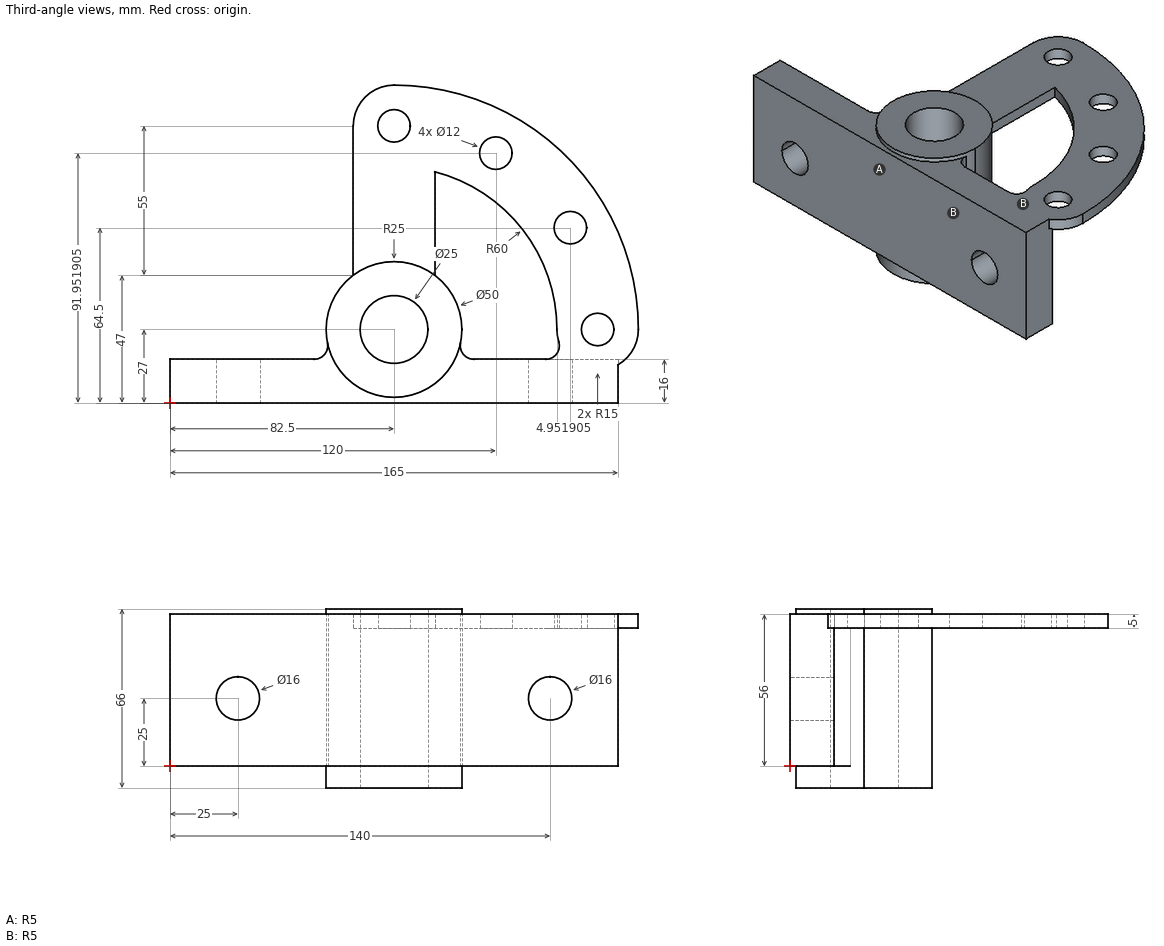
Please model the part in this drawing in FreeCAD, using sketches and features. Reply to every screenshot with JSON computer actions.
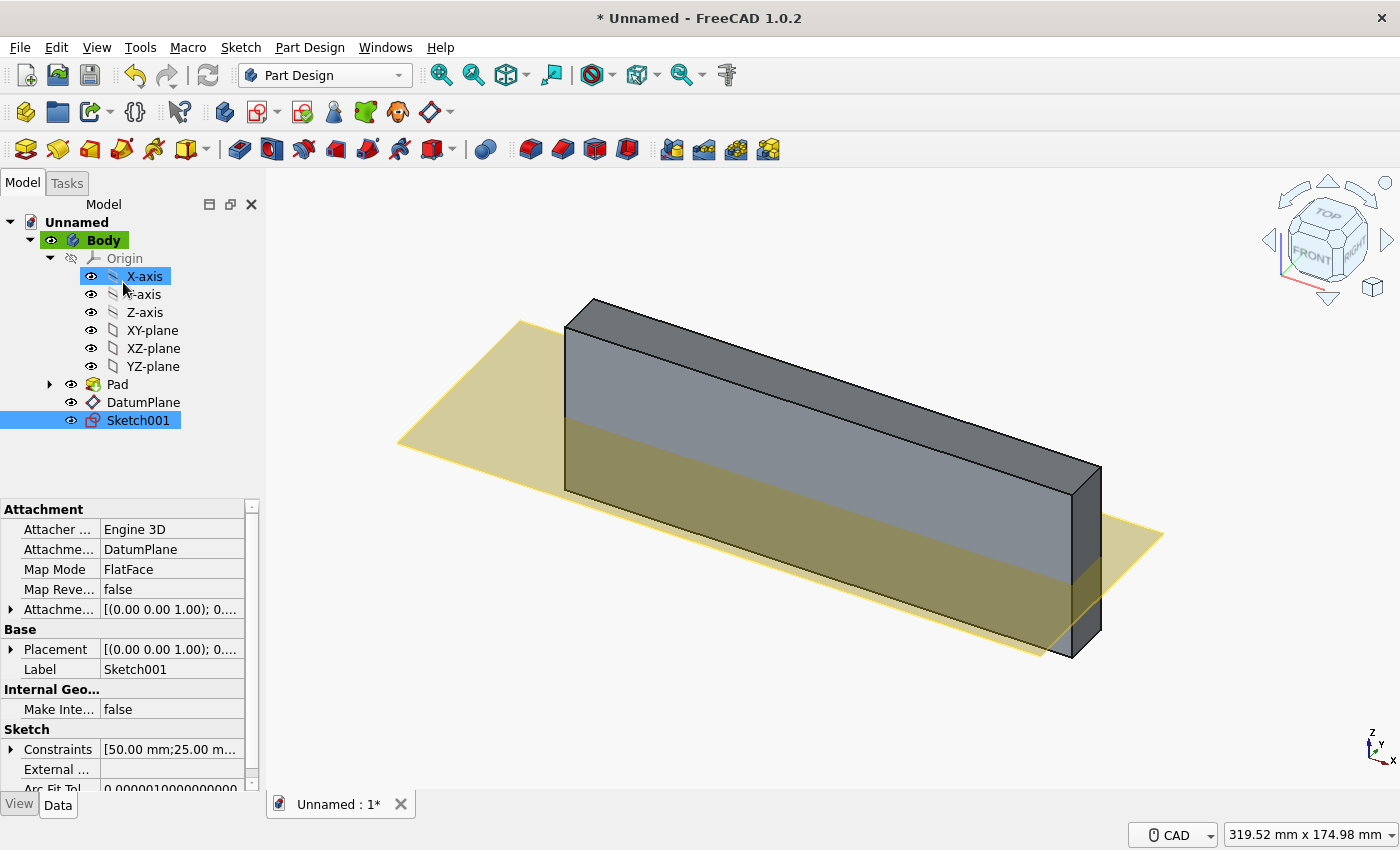
{"action": "left_click", "coordinate": [26, 150]}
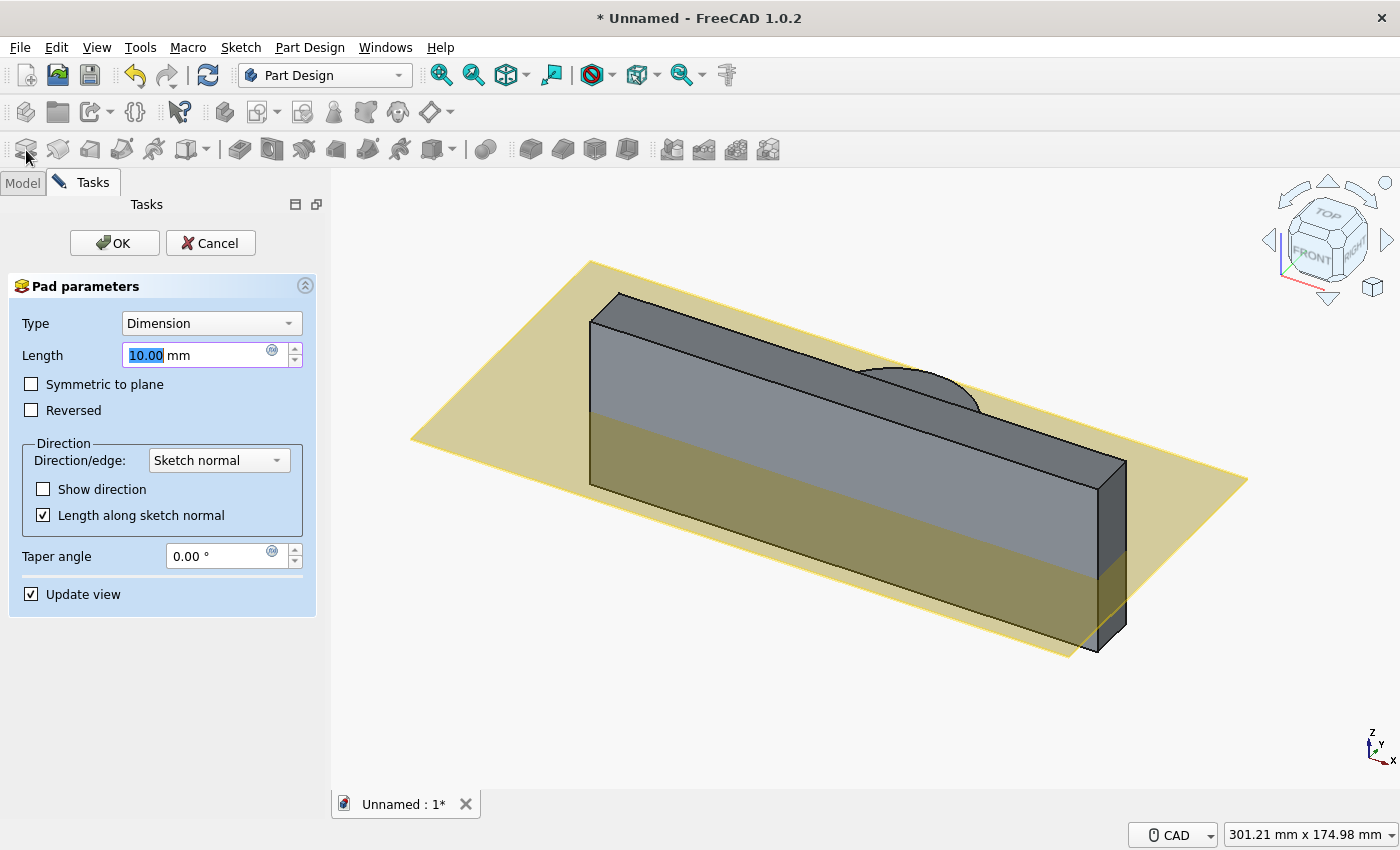
{"action": "type", "text": "66"}
{"action": "key", "text": "Tab"}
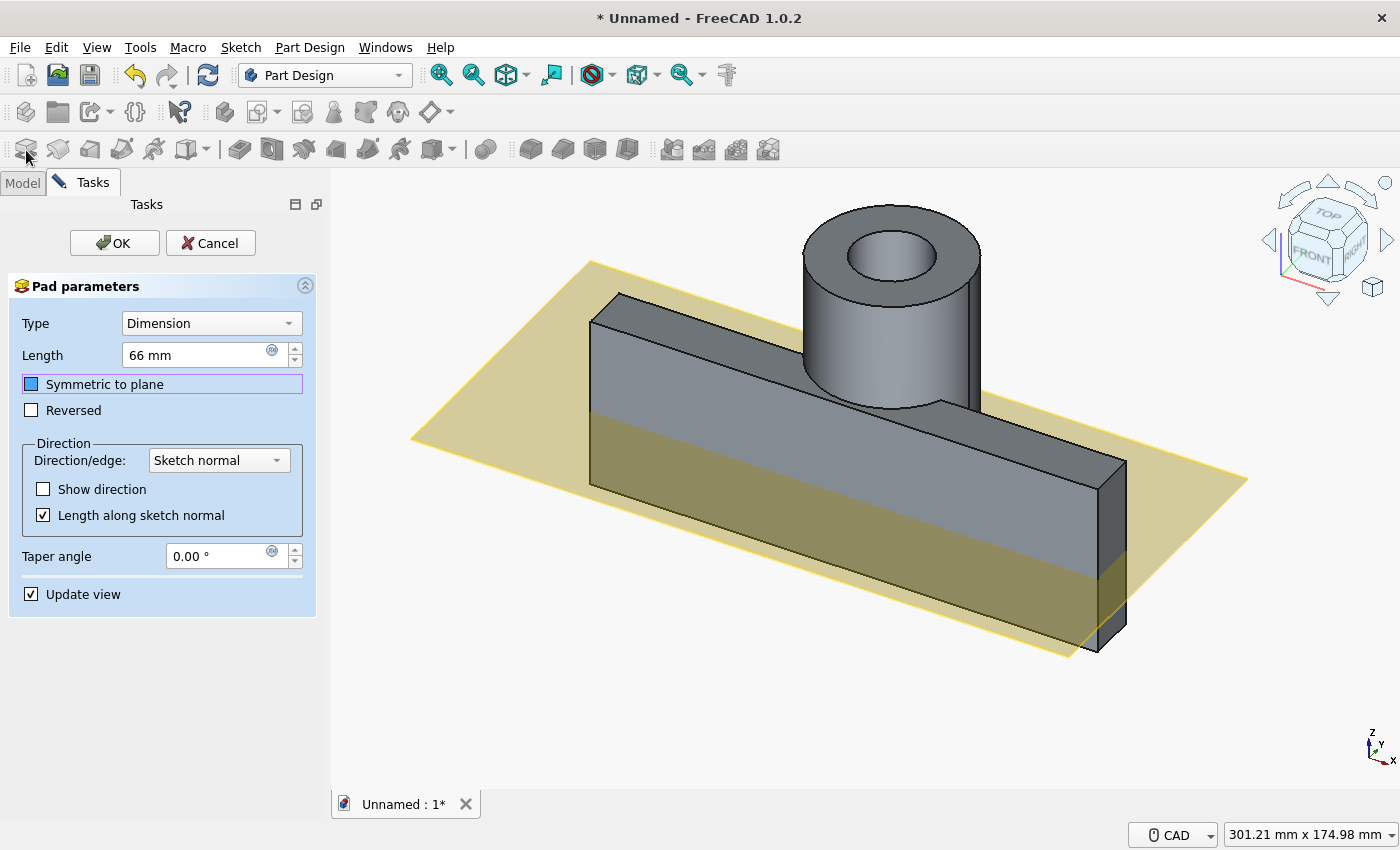
{"action": "left_click", "coordinate": [30, 384]}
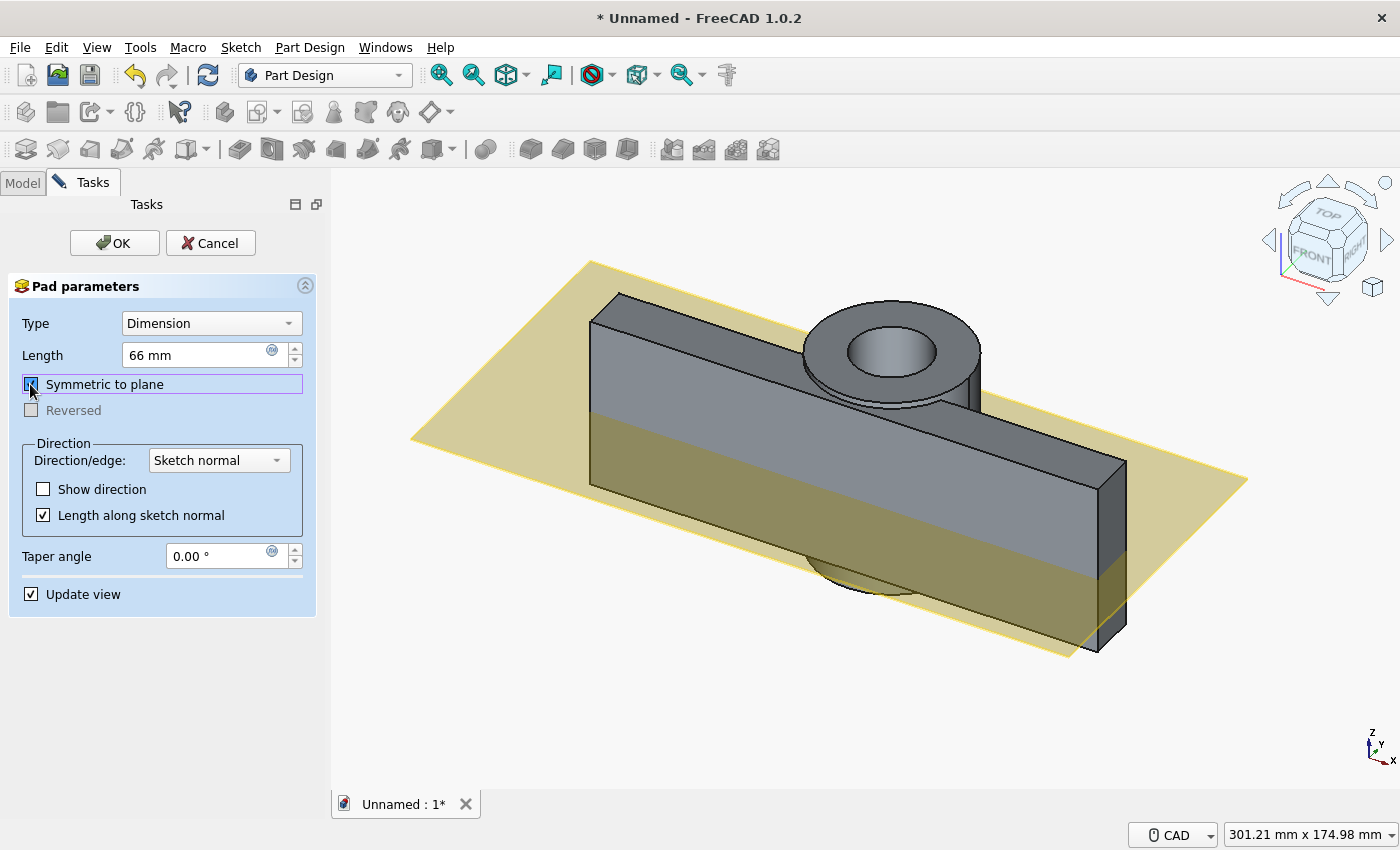
{"action": "left_click", "coordinate": [115, 243]}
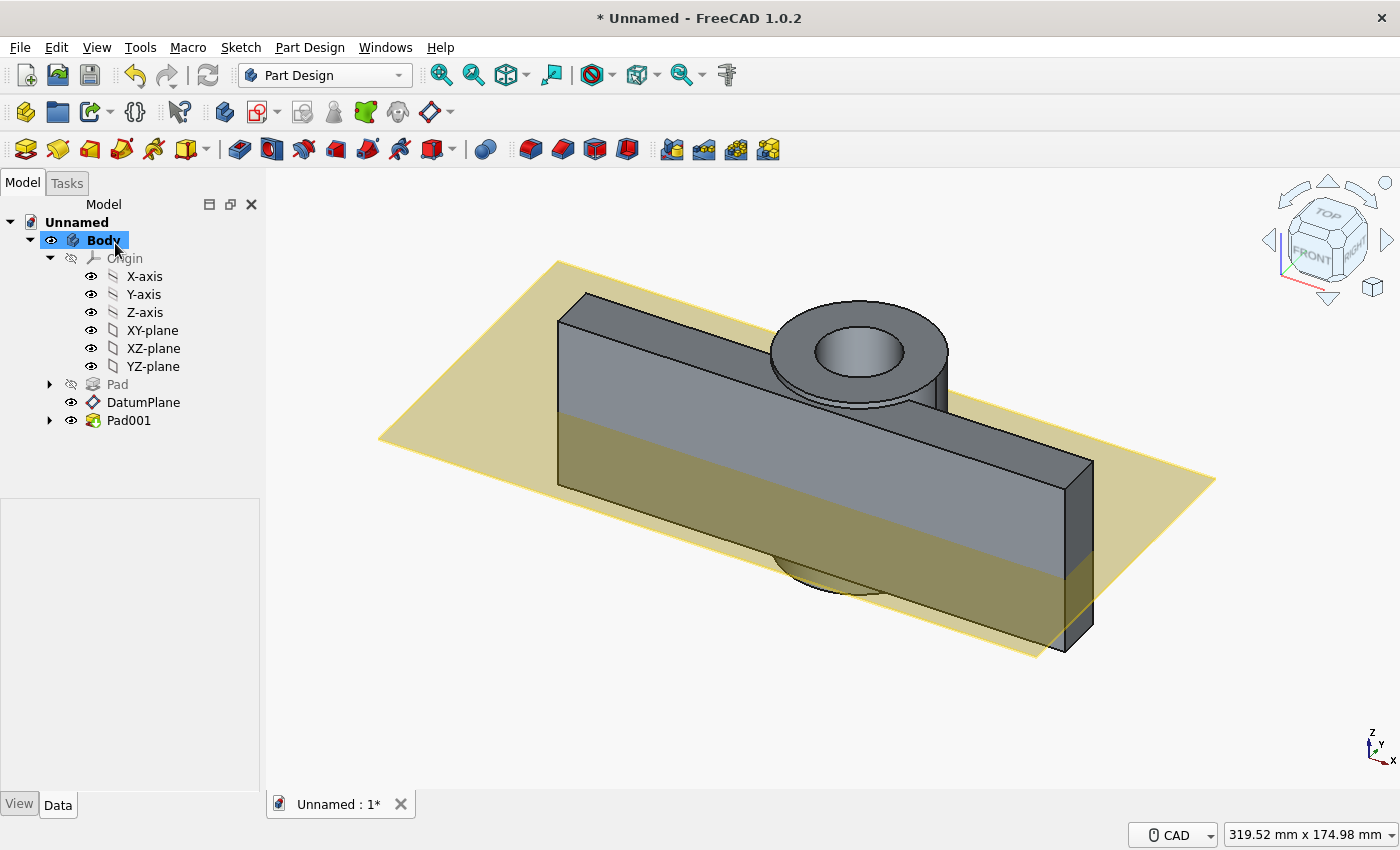
{"action": "left_click", "coordinate": [116, 402]}
{"action": "key", "text": "space"}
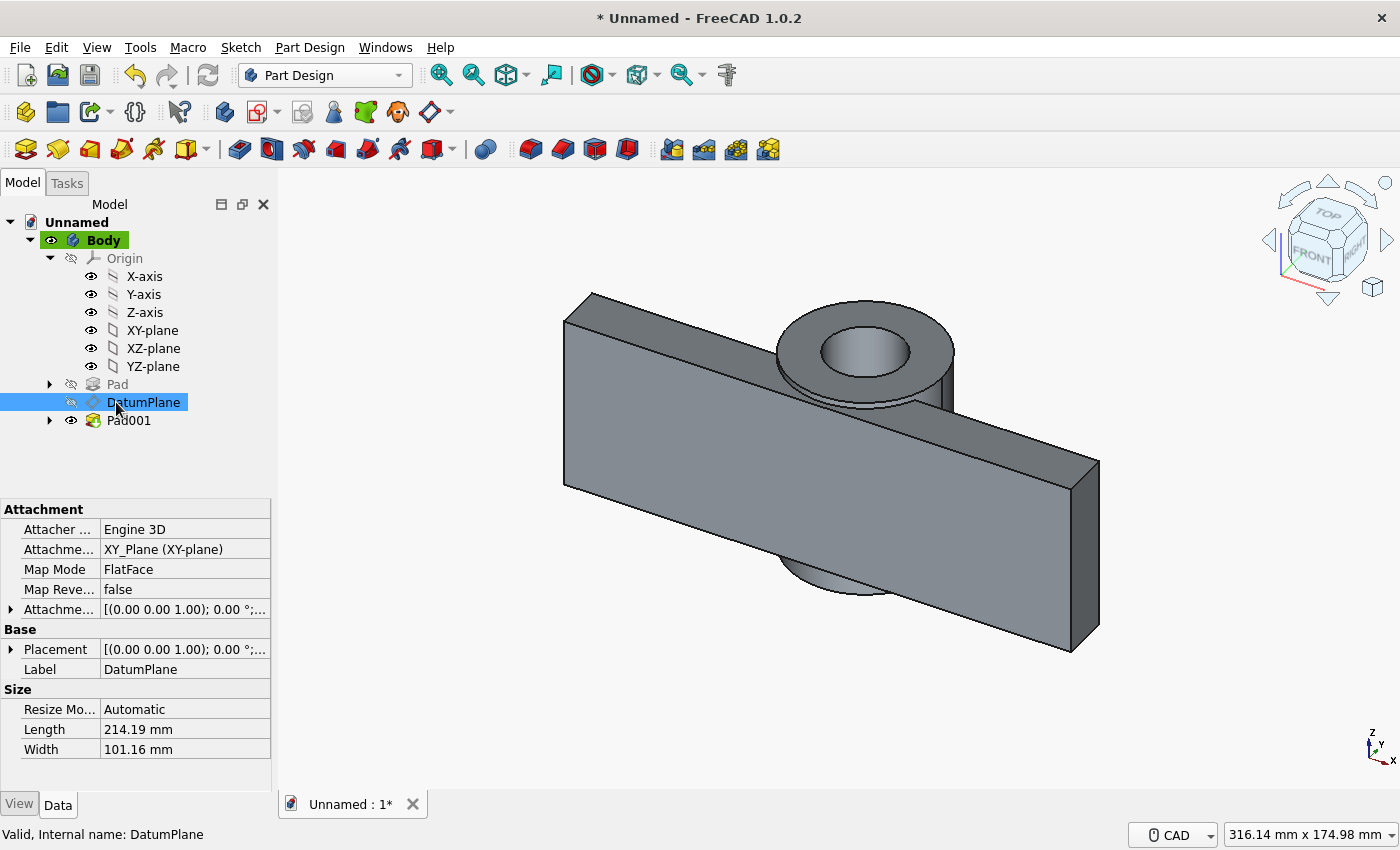
{"action": "left_click", "coordinate": [935, 340]}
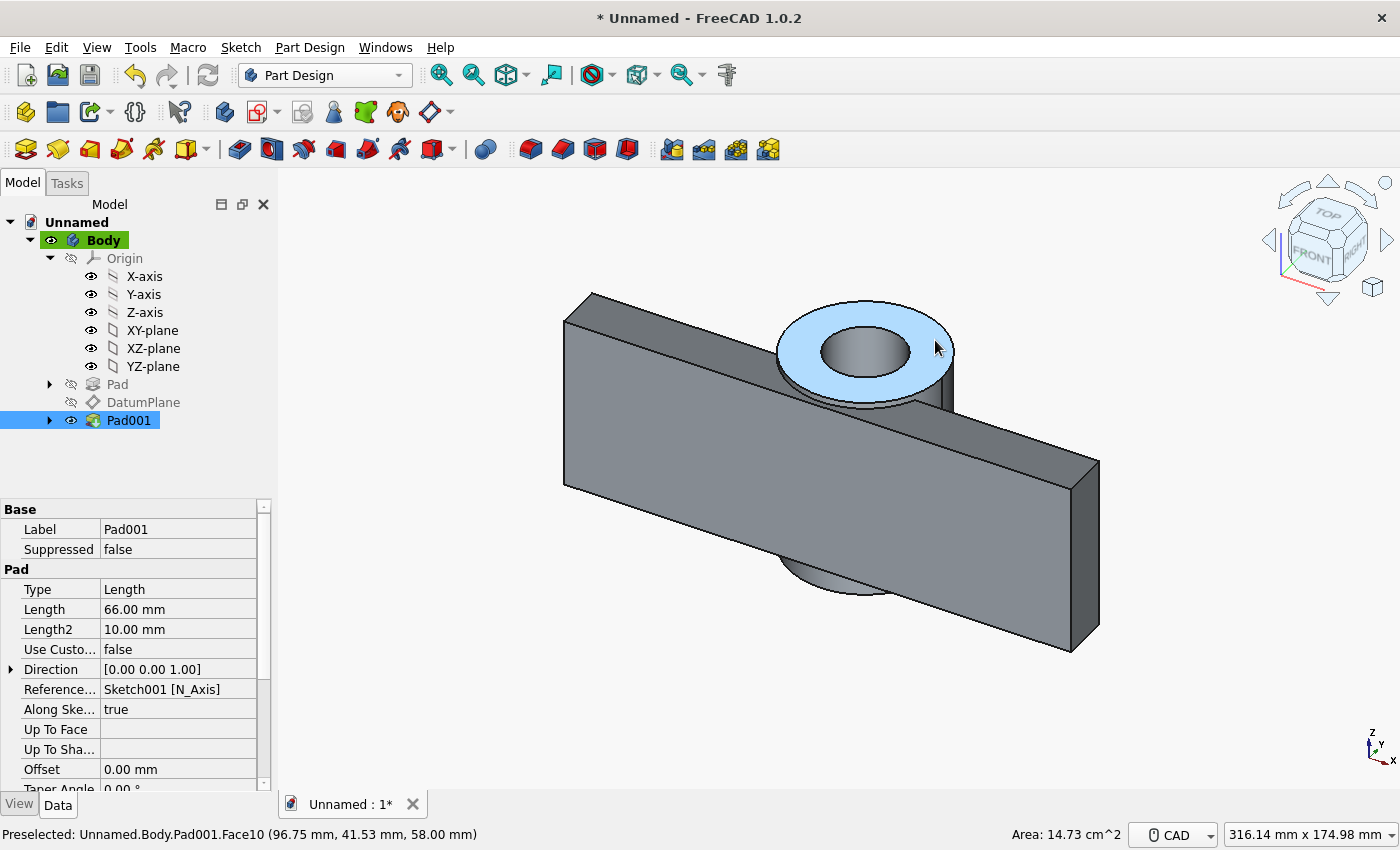
{"action": "left_click", "coordinate": [258, 112]}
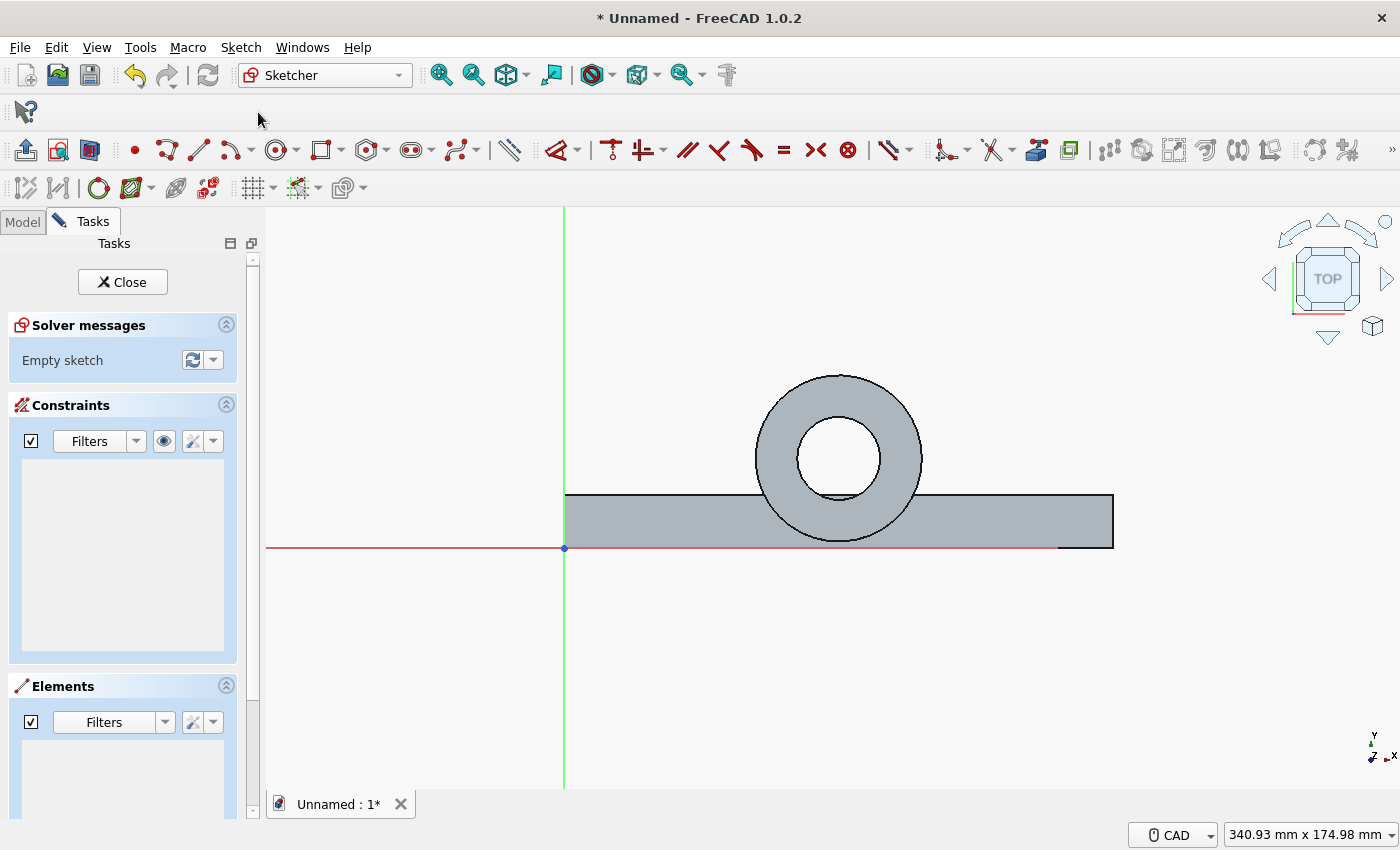
{"action": "scroll", "coordinate": [863, 445], "scroll_direction": "up", "scroll_amount": 7}